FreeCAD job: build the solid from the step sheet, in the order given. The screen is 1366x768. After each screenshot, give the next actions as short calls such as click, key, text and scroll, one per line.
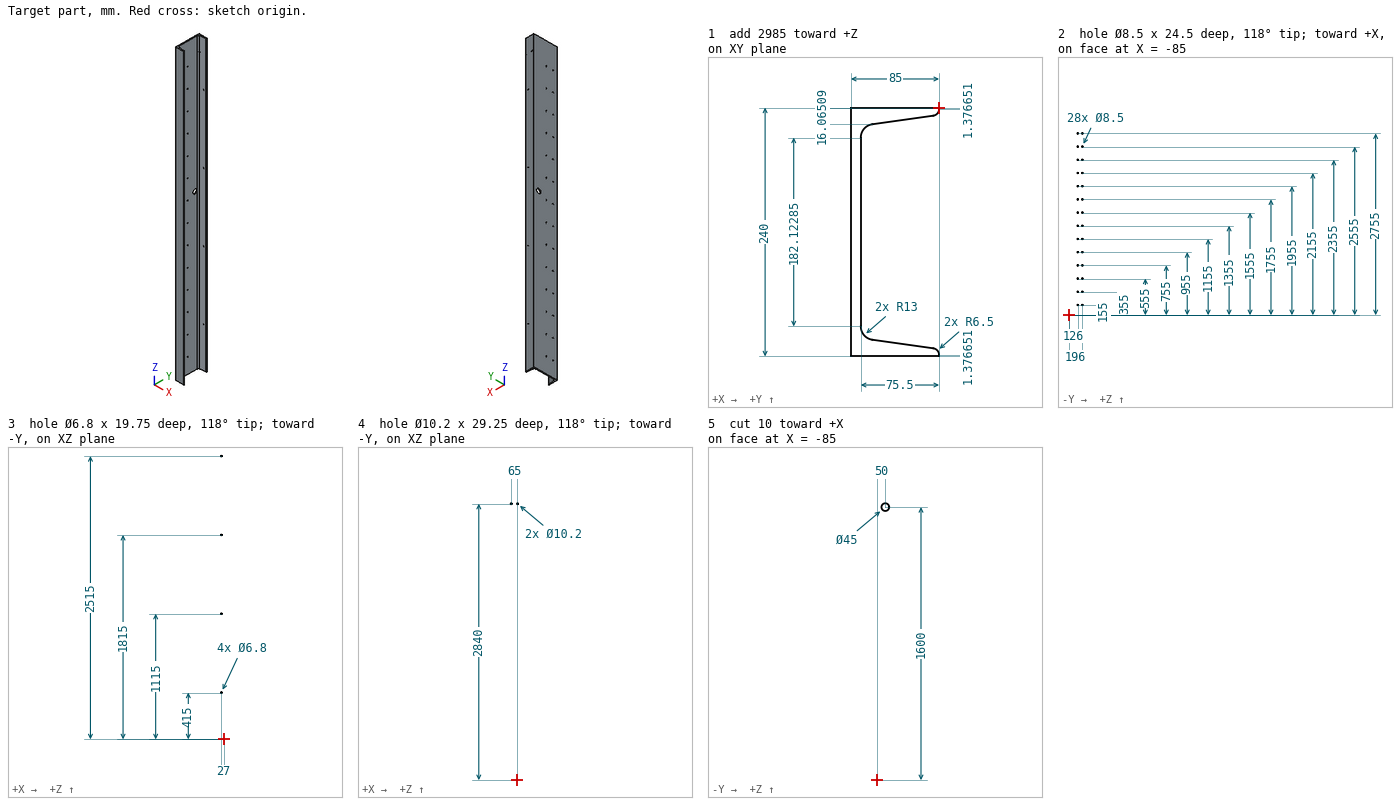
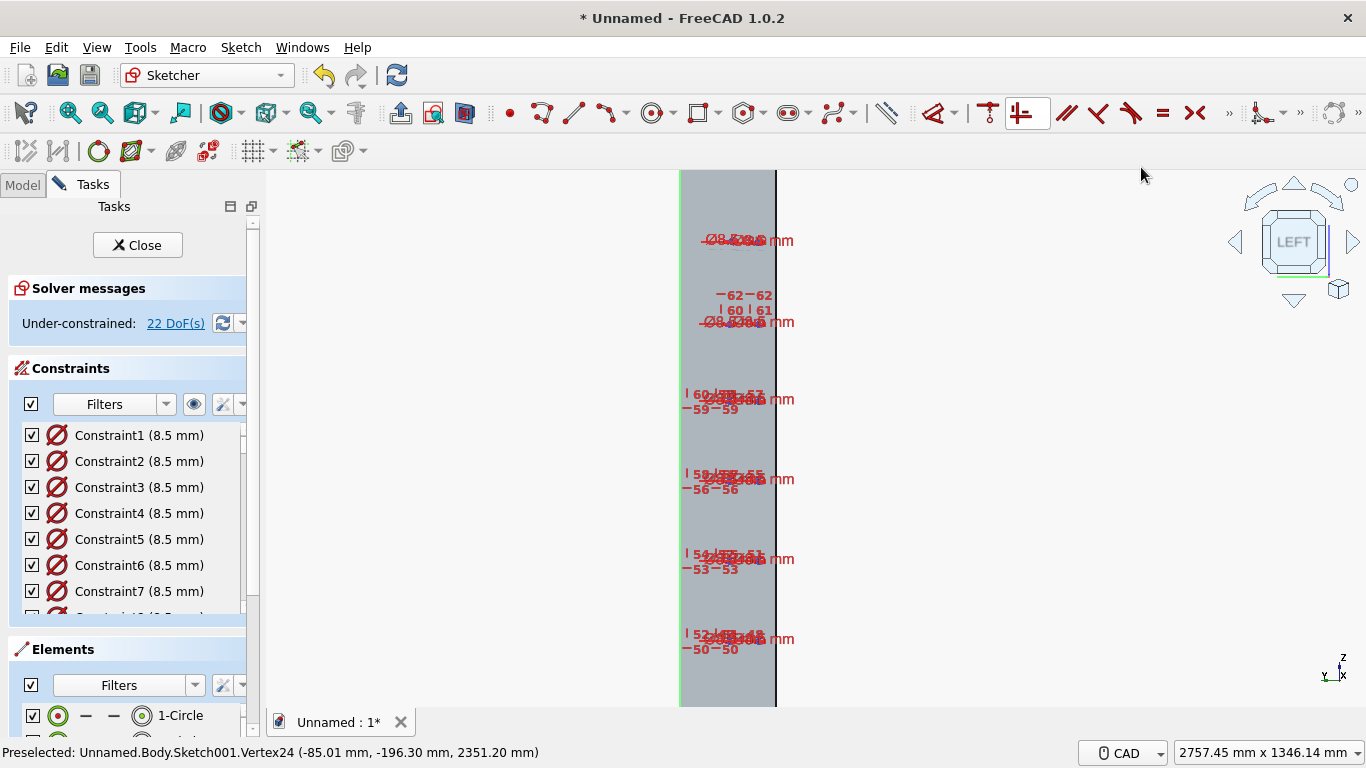
click(758, 324)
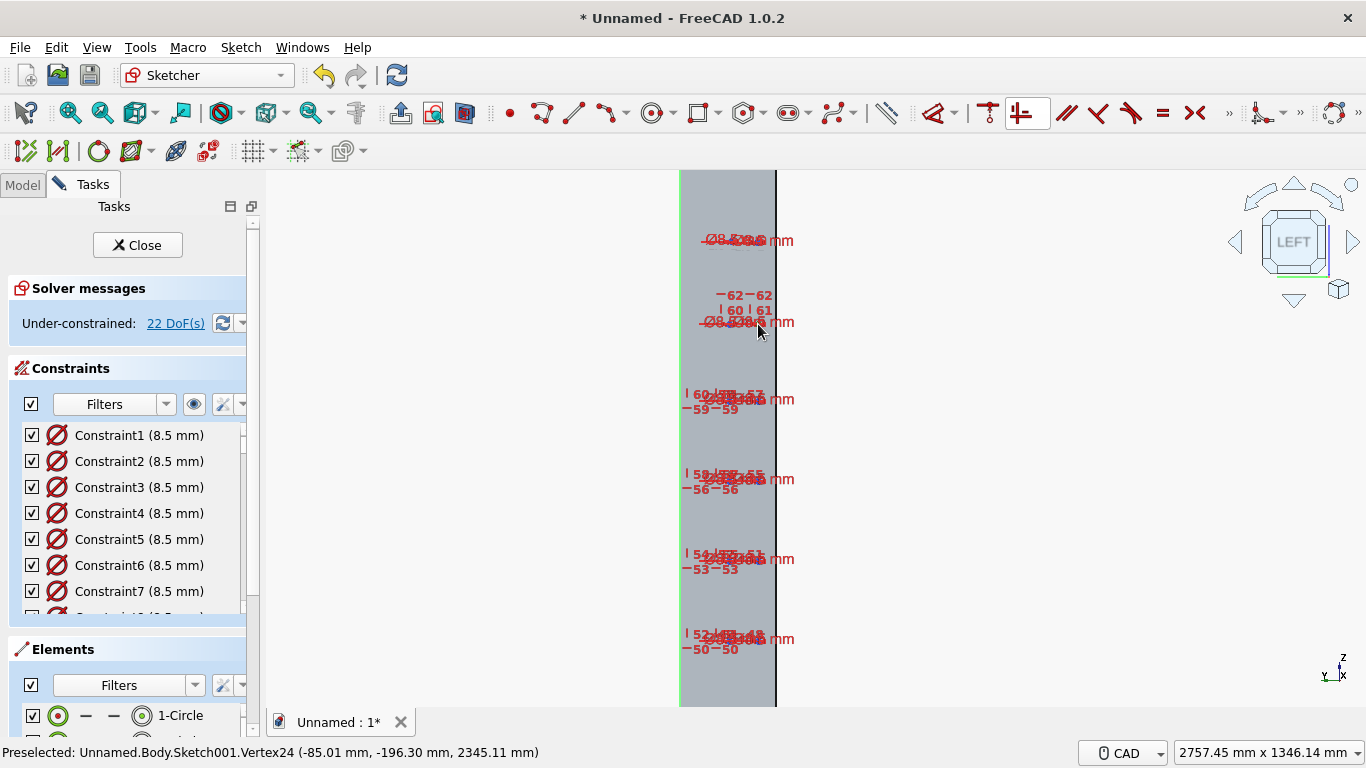
click(758, 243)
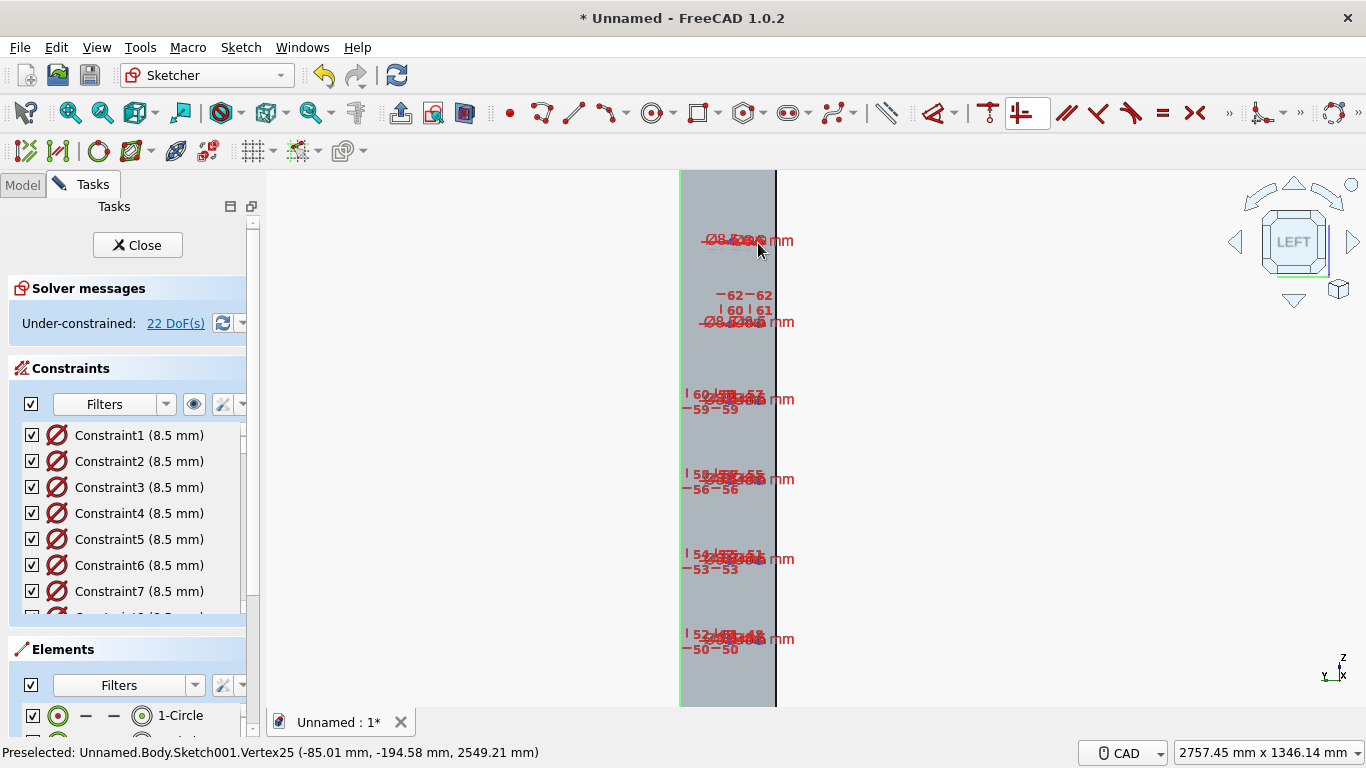
click(1044, 114)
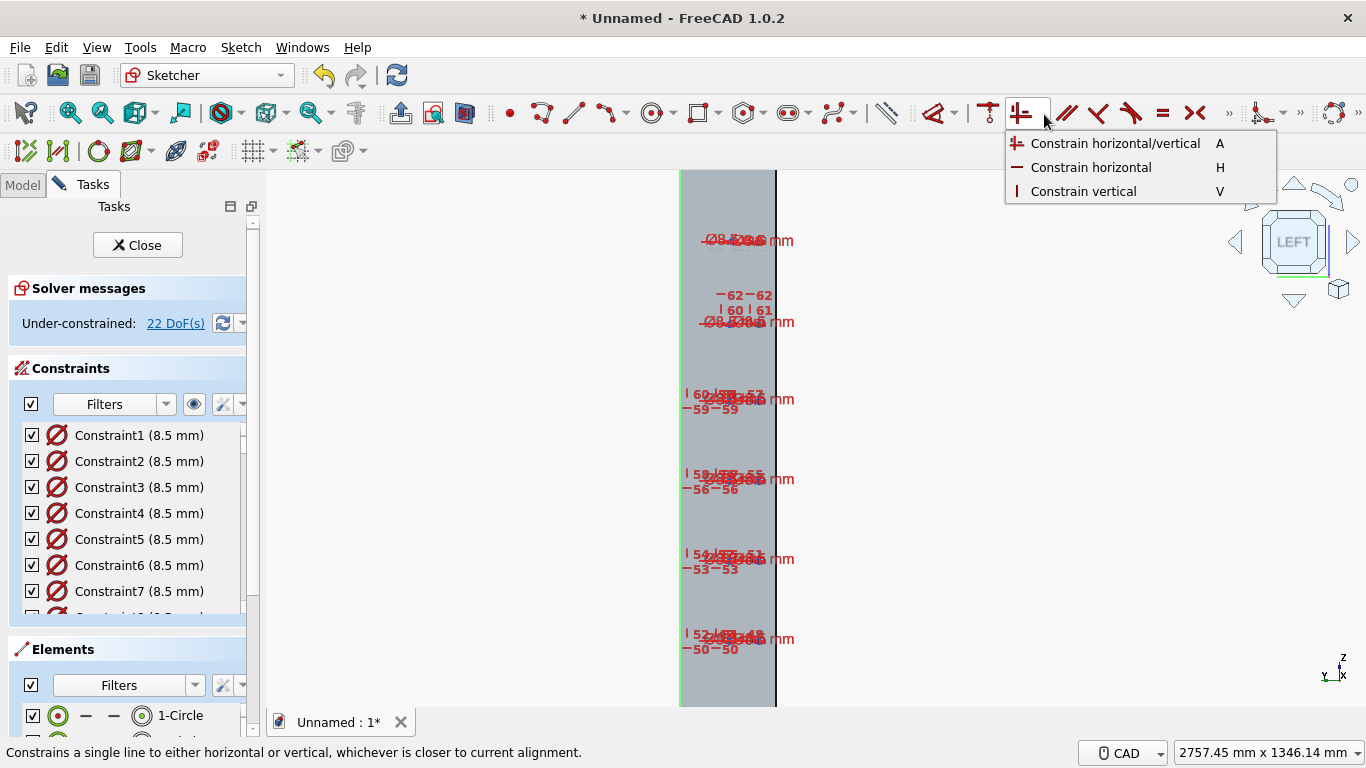
click(1141, 191)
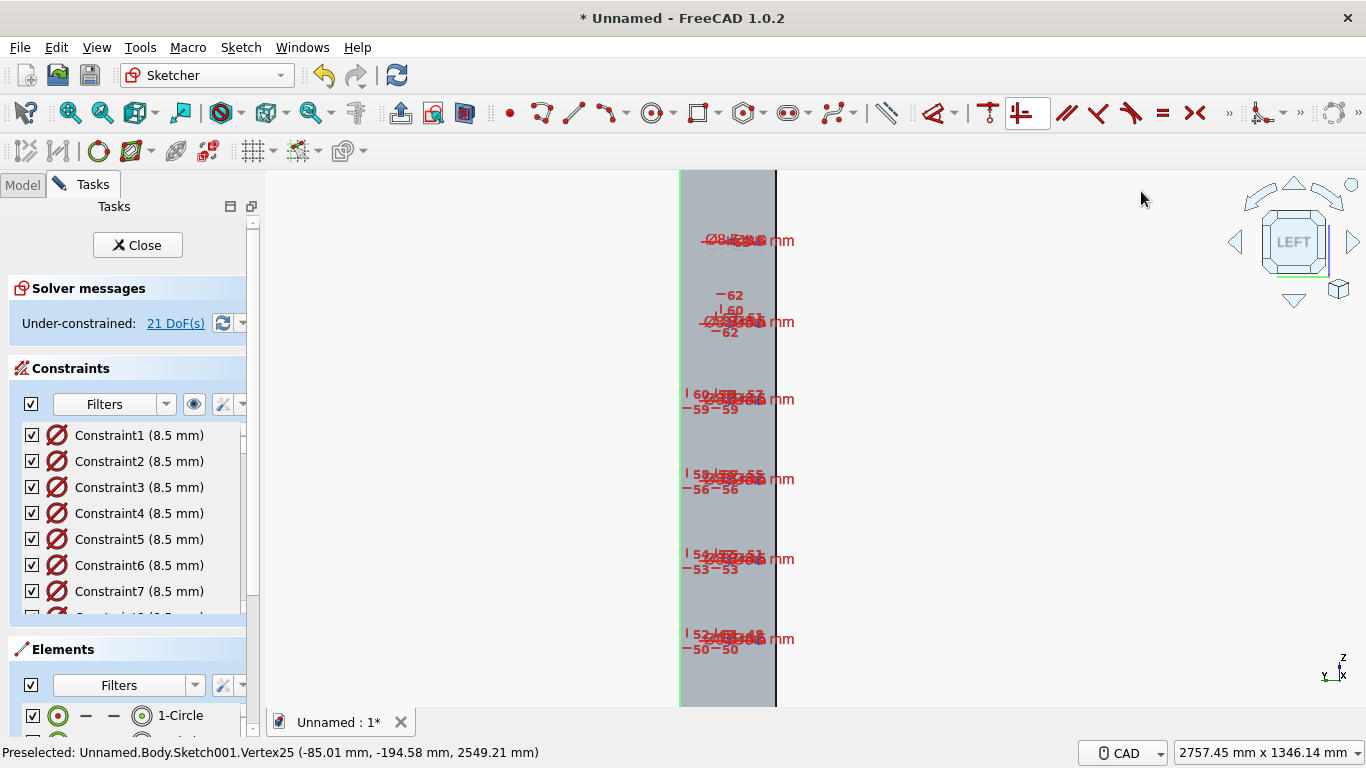
click(729, 324)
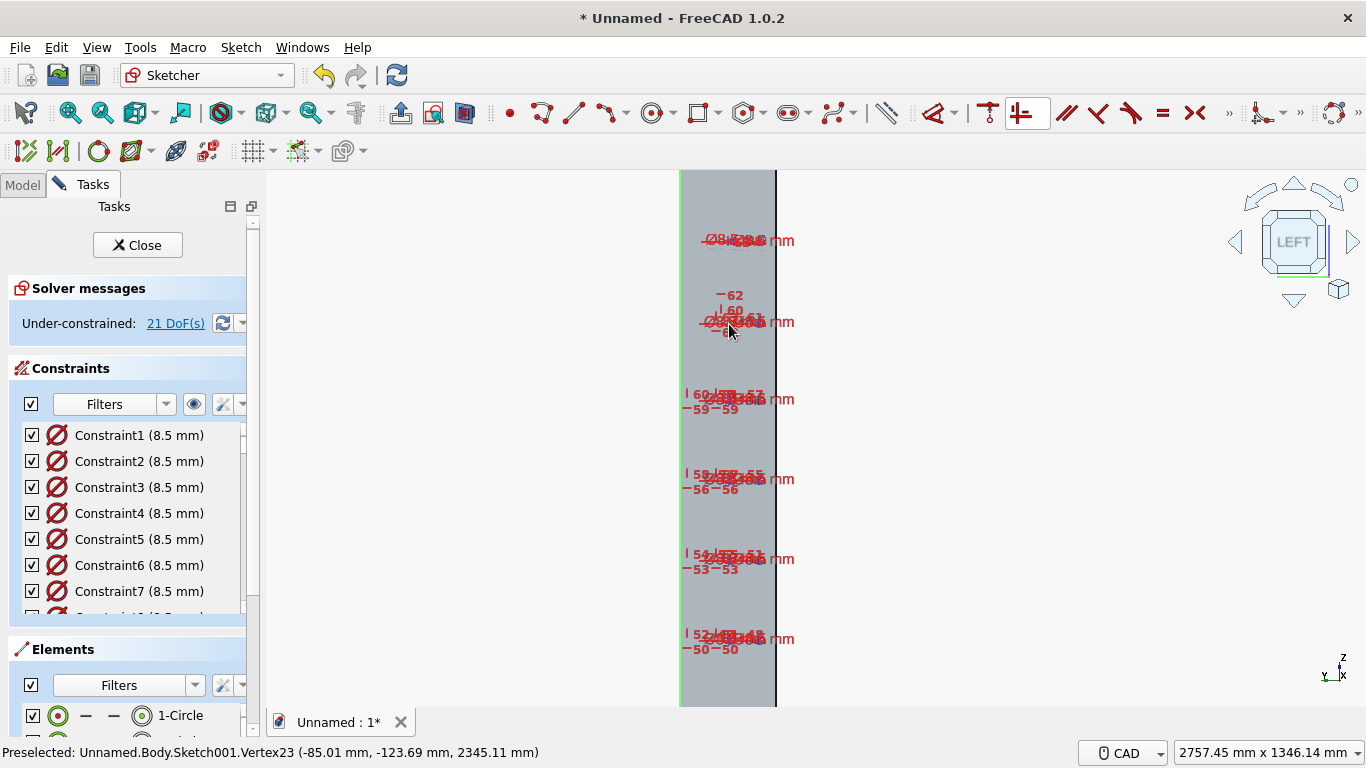
scroll(731, 242, up, 4)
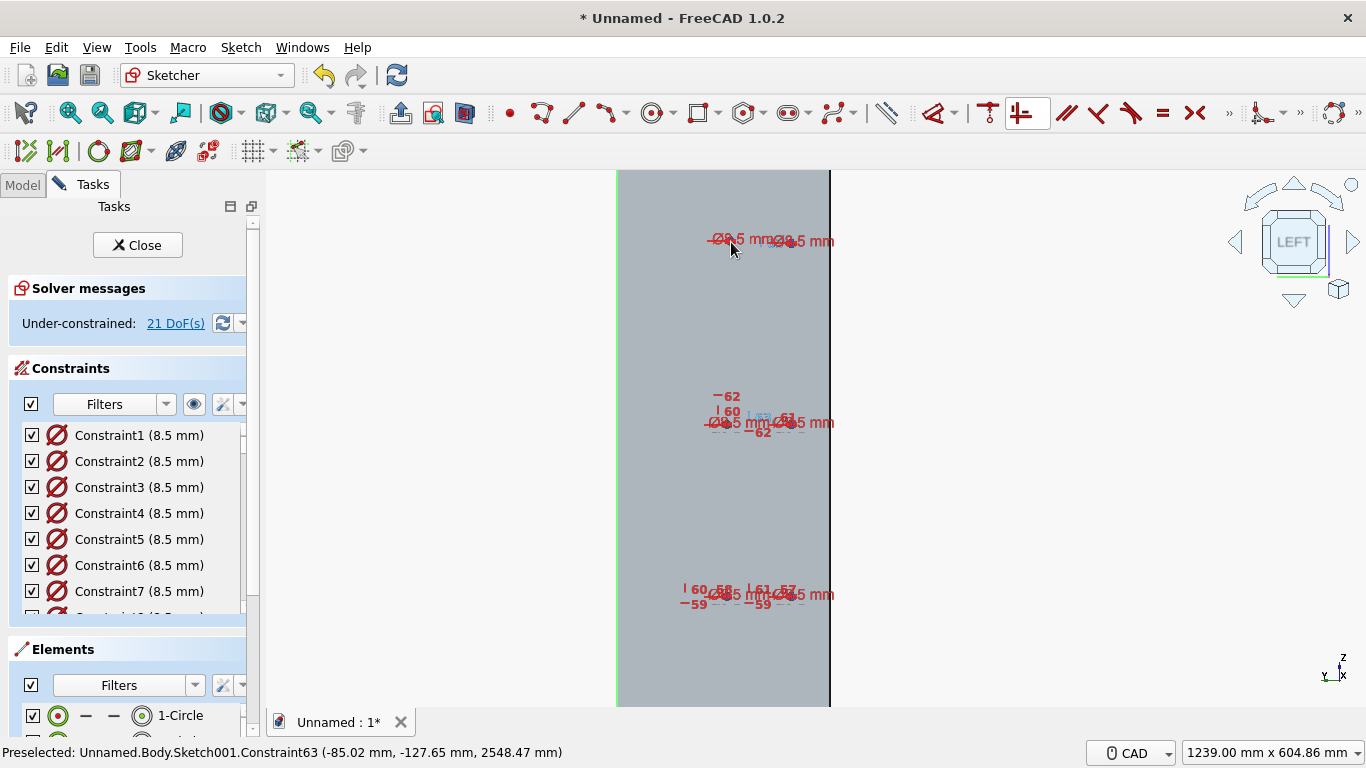
click(731, 241)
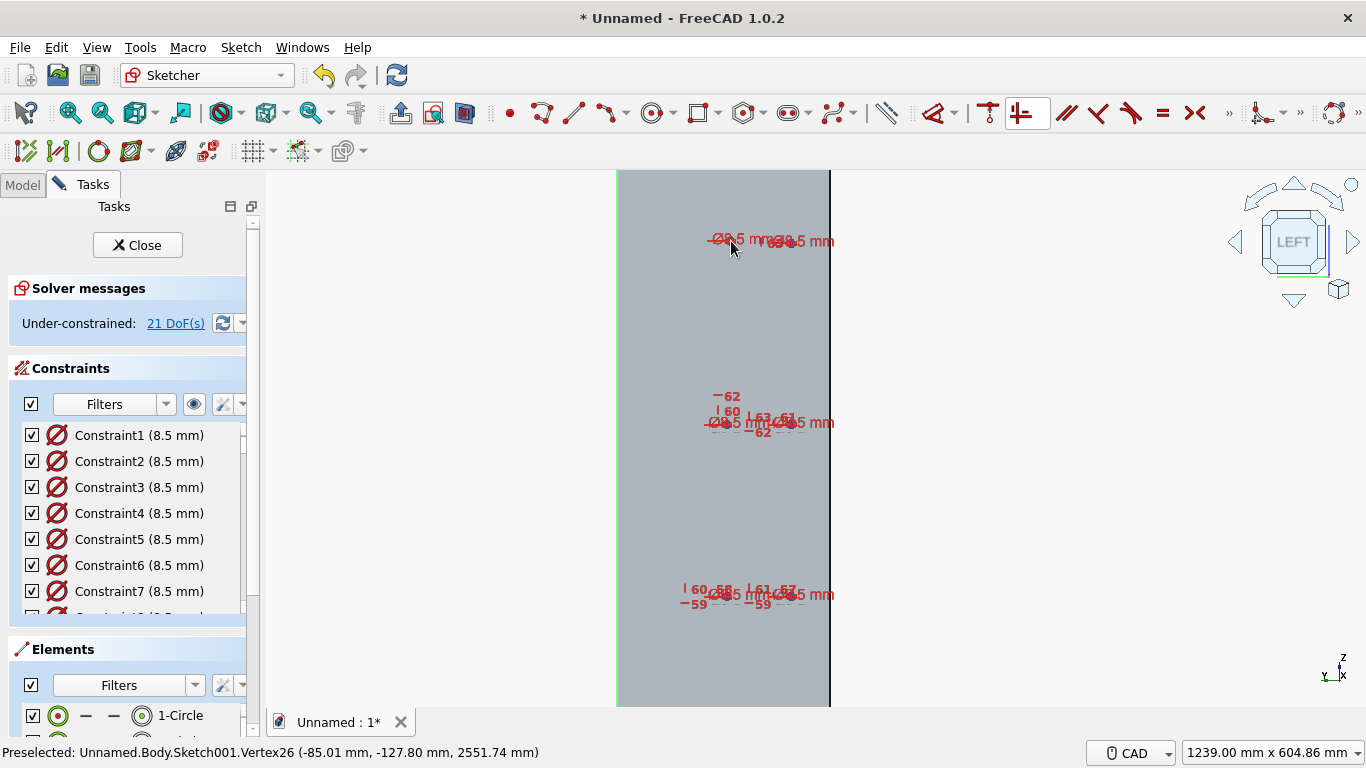
click(1044, 114)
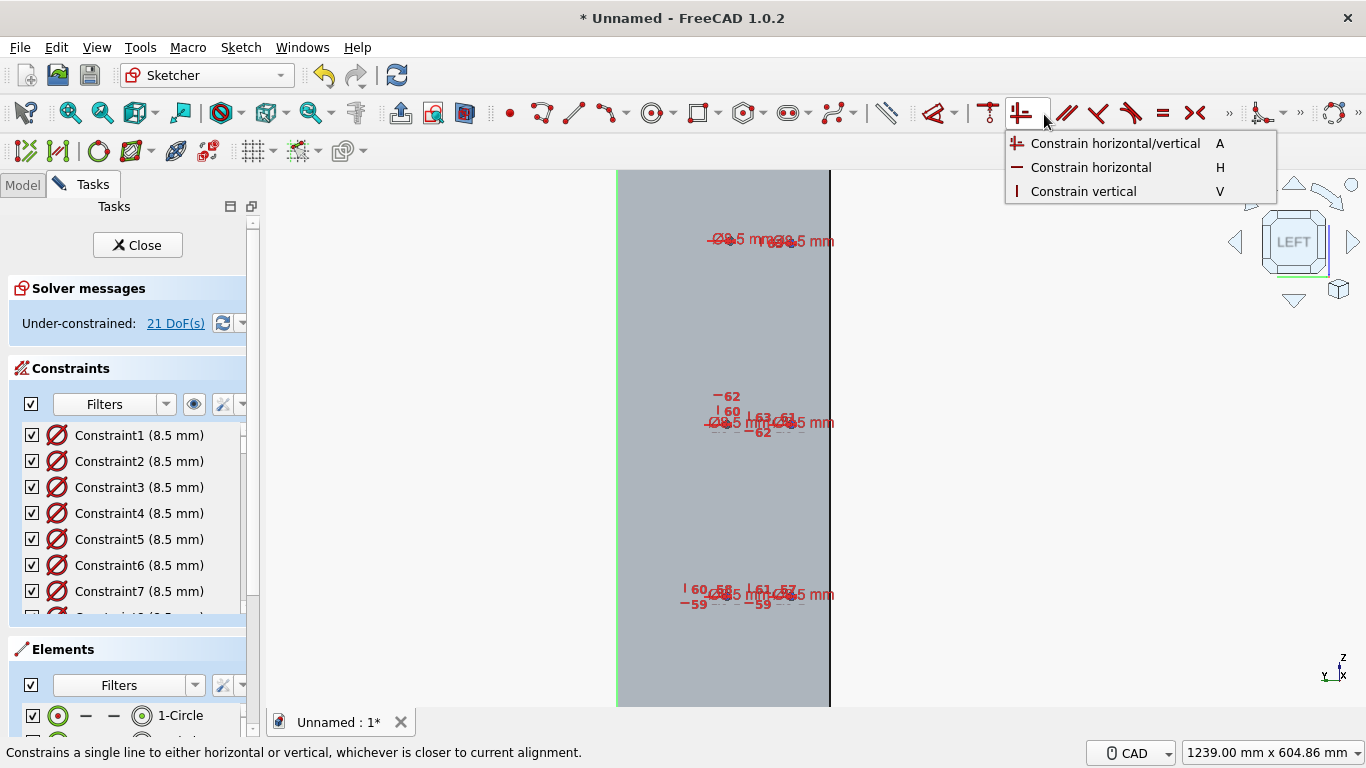
click(1141, 191)